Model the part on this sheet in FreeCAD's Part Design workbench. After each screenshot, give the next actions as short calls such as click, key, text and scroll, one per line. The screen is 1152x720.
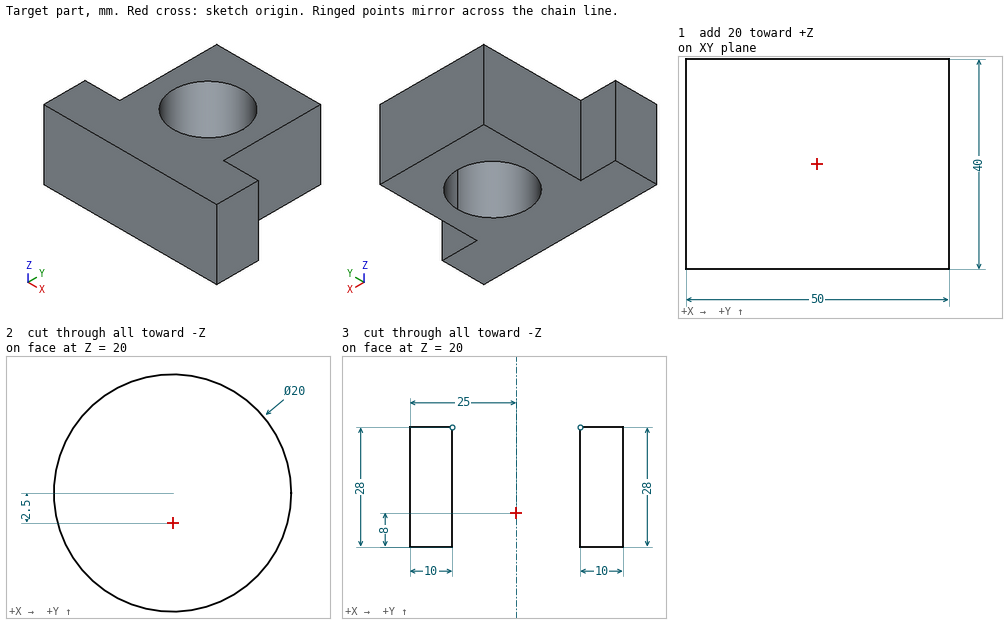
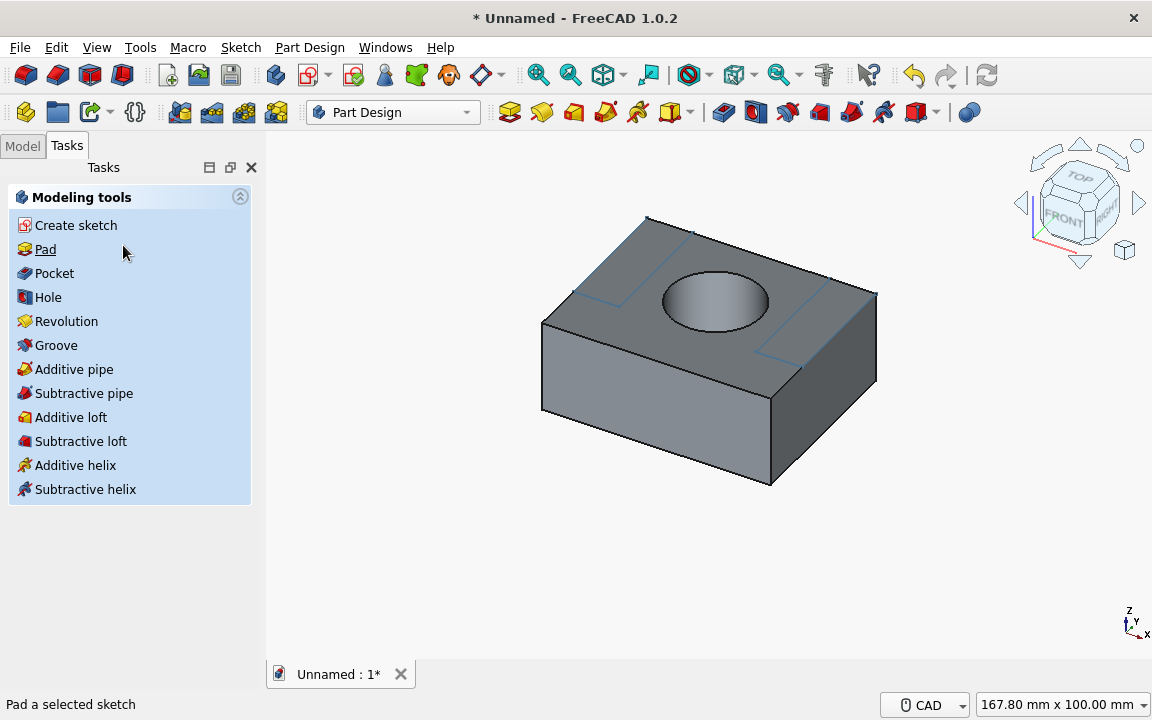
click(724, 112)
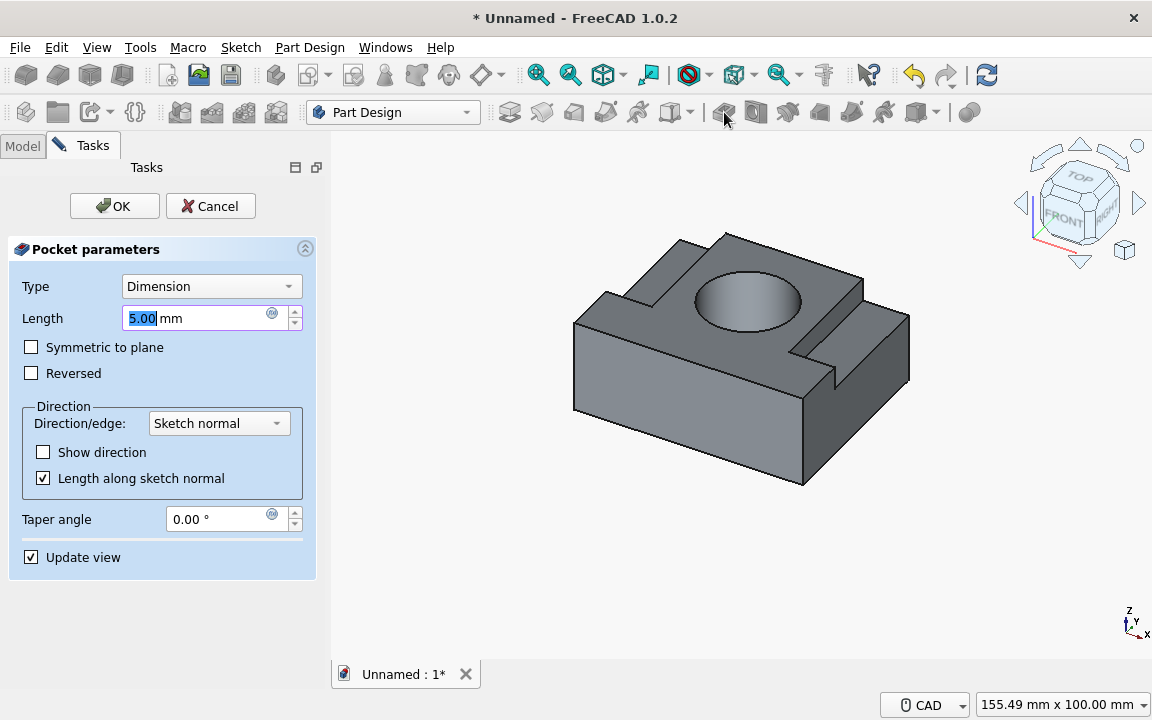
click(212, 286)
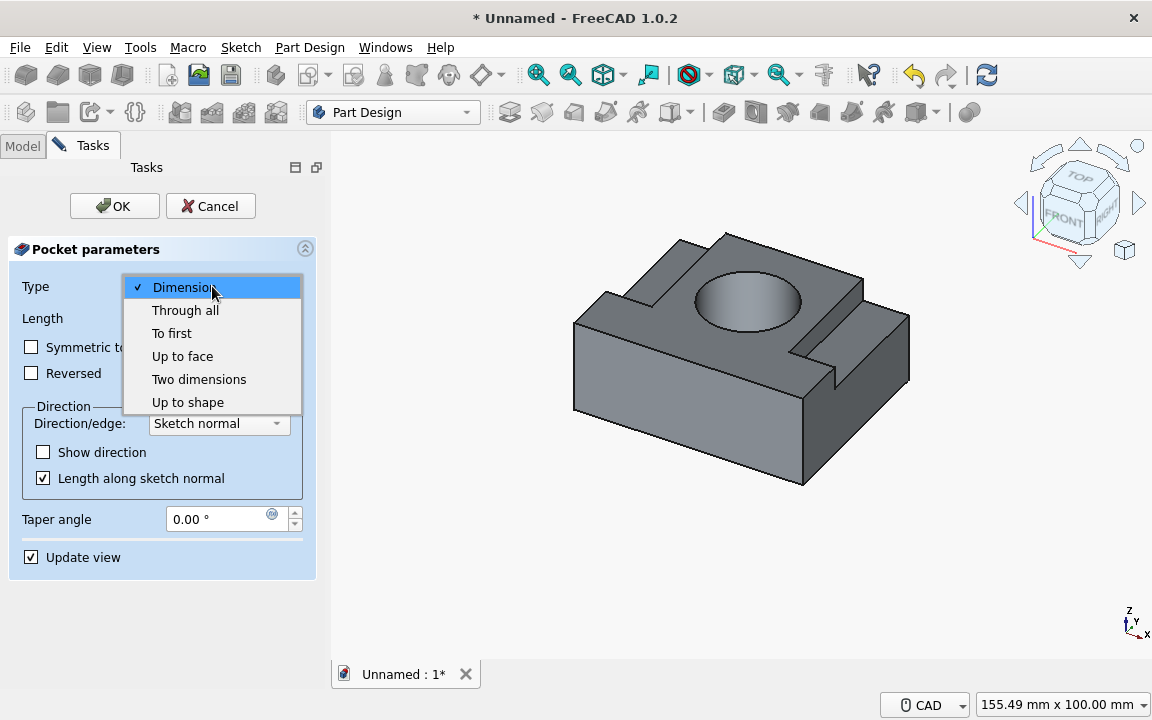
click(212, 310)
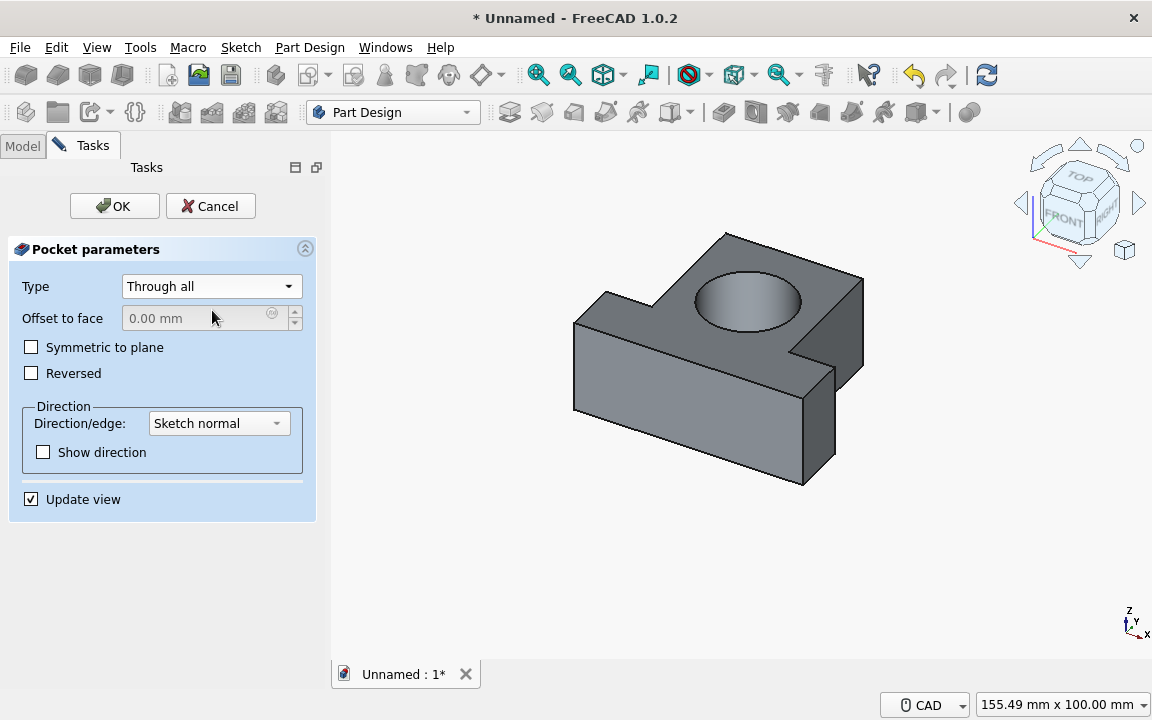
click(115, 206)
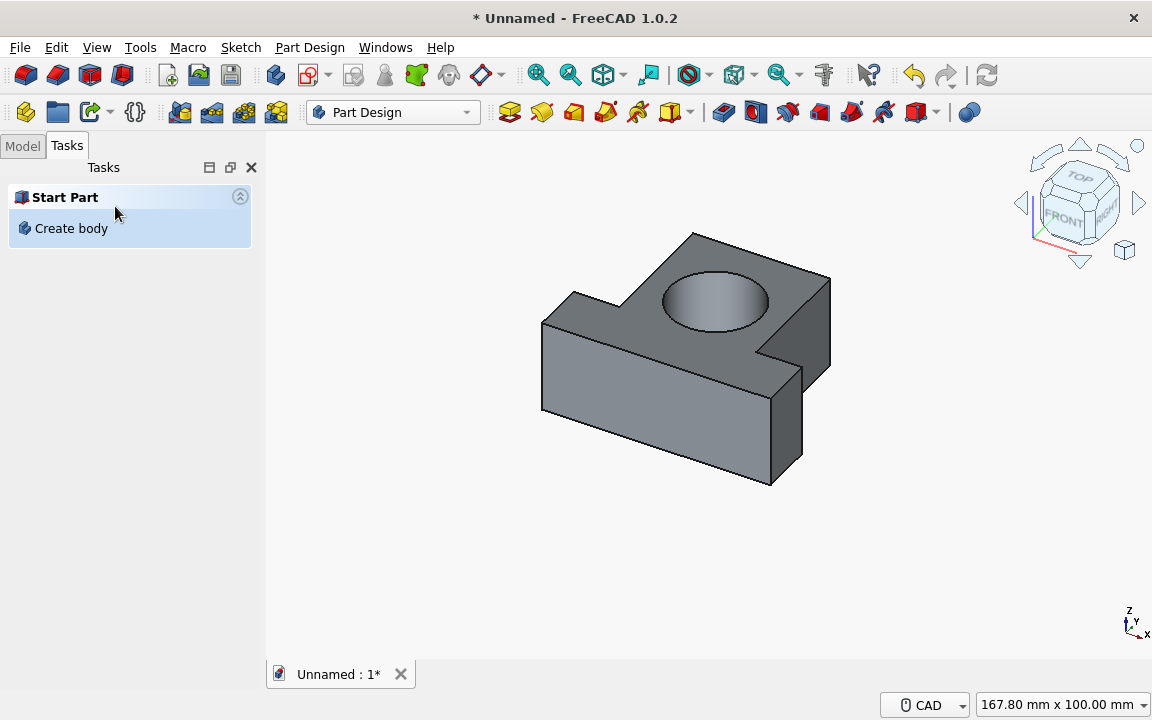
key(0)